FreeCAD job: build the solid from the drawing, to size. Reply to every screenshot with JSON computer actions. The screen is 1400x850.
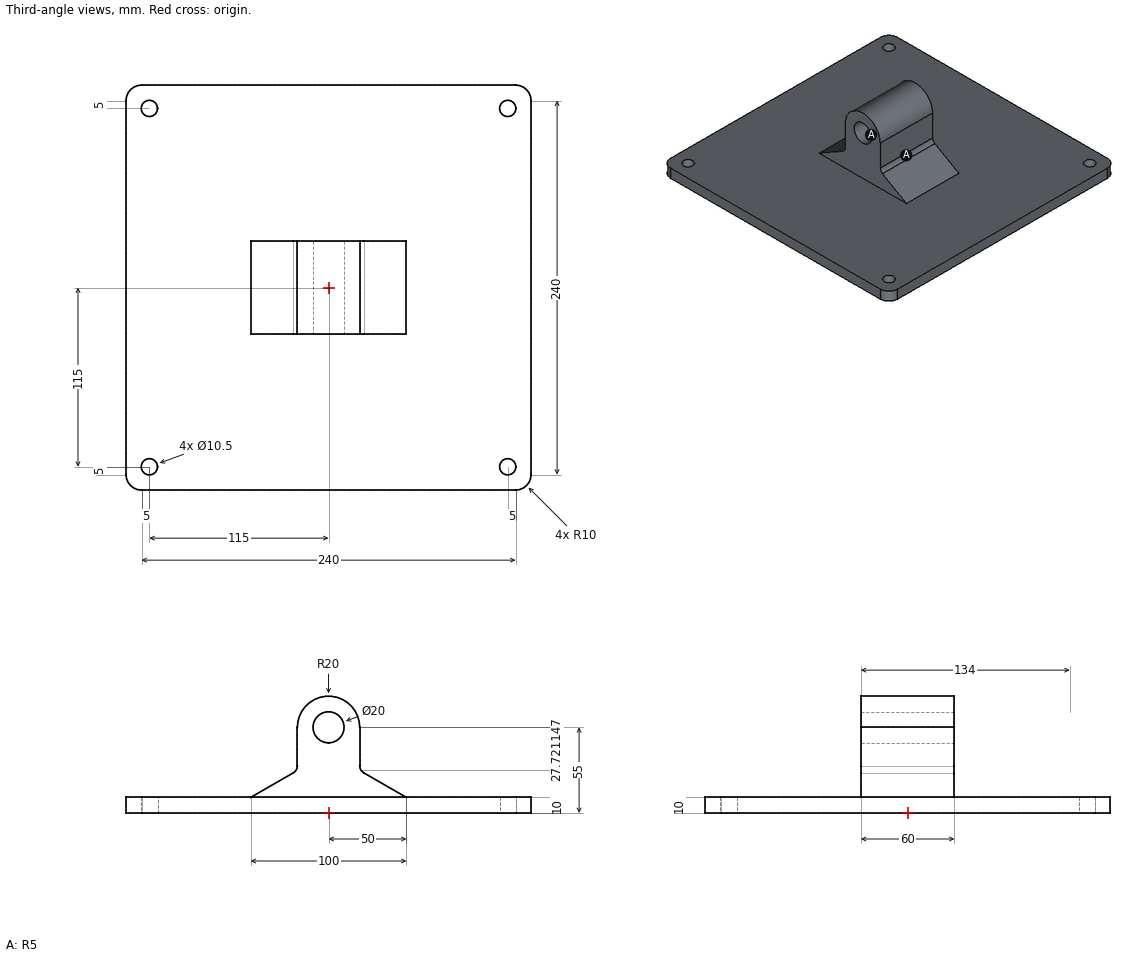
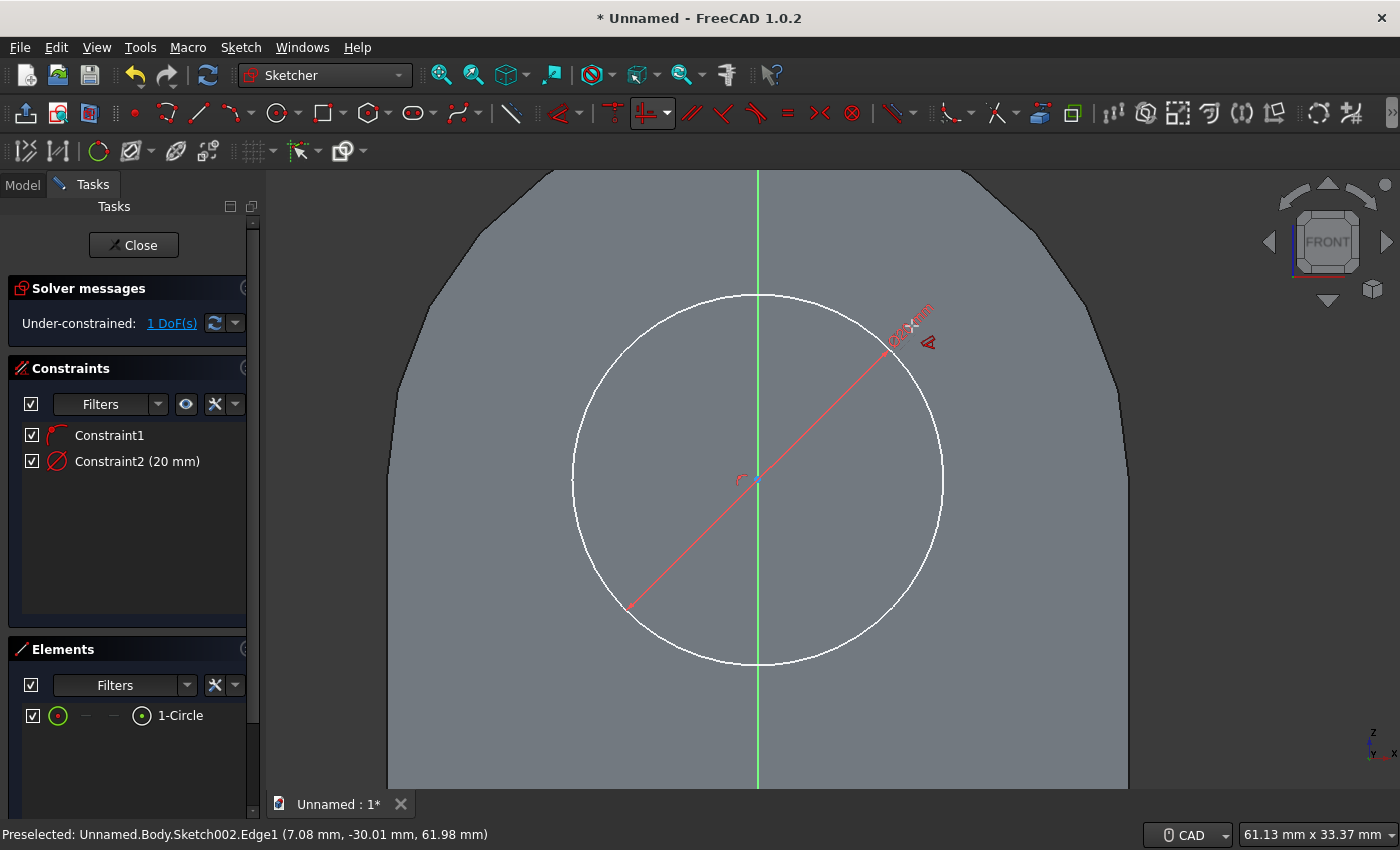
{"action": "left_click", "coordinate": [758, 480]}
{"action": "left_click", "coordinate": [792, 621]}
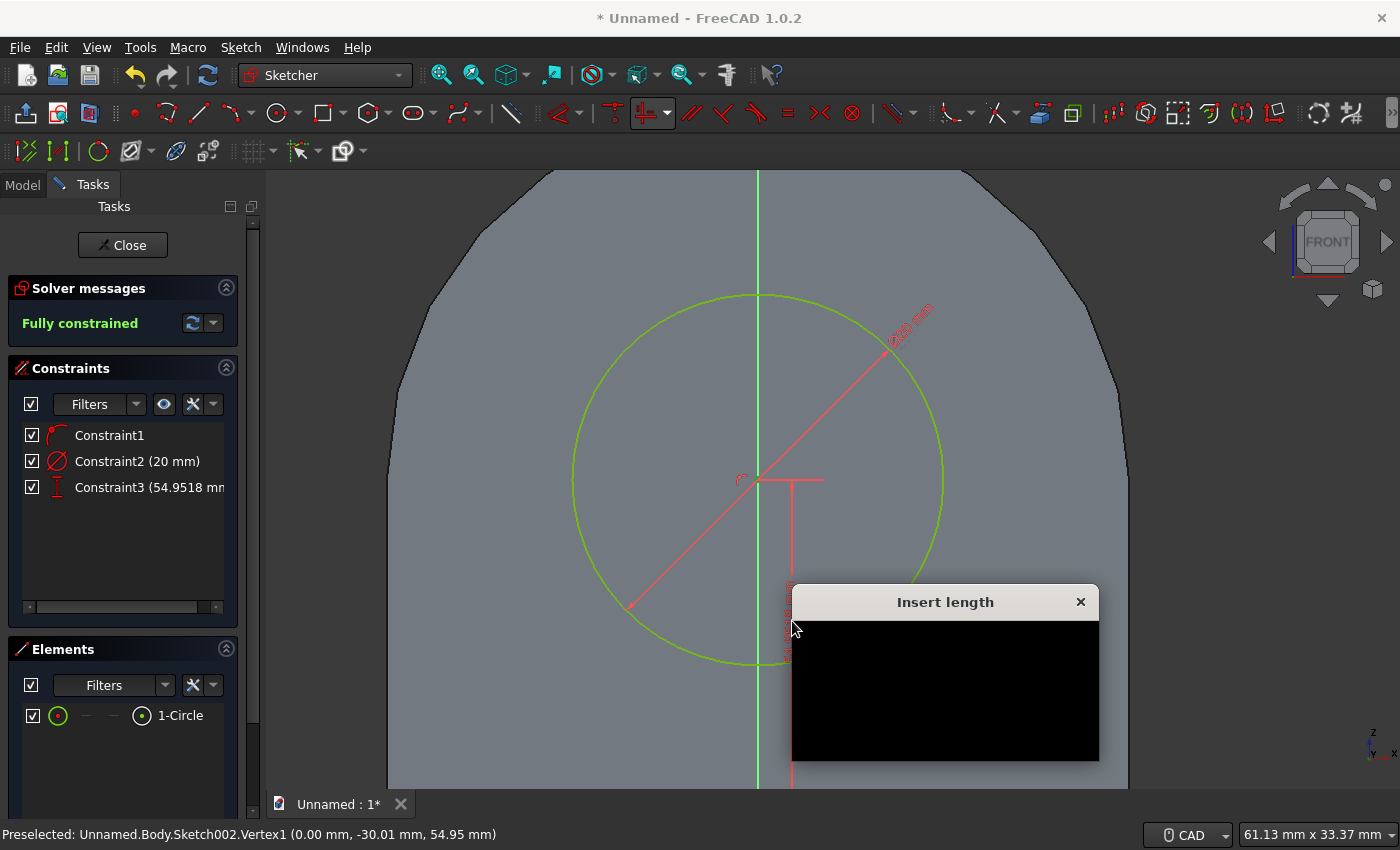
{"action": "type", "text": "55"}
{"action": "key", "text": "Return"}
{"action": "key", "text": "Escape"}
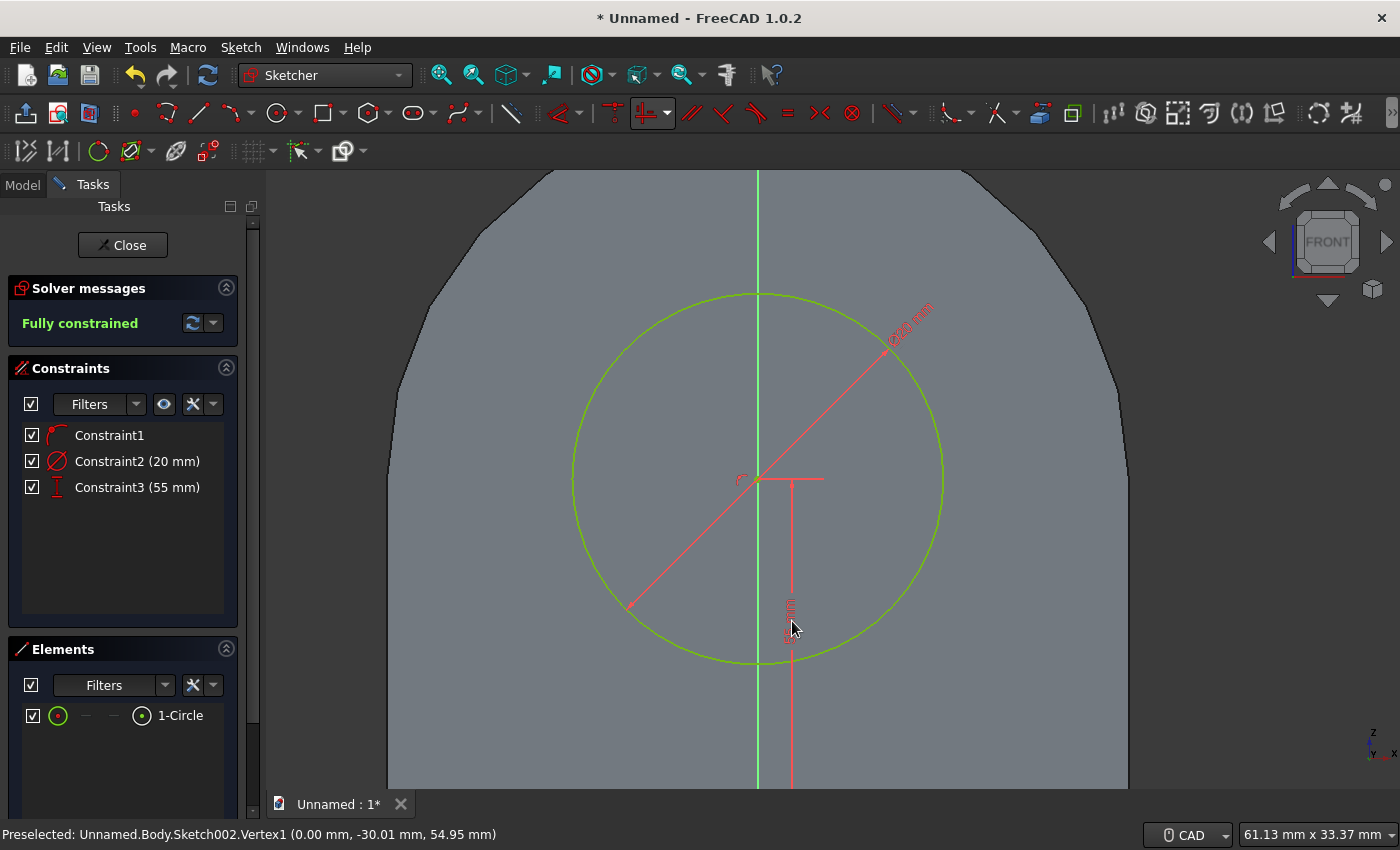
{"action": "left_click", "coordinate": [123, 245]}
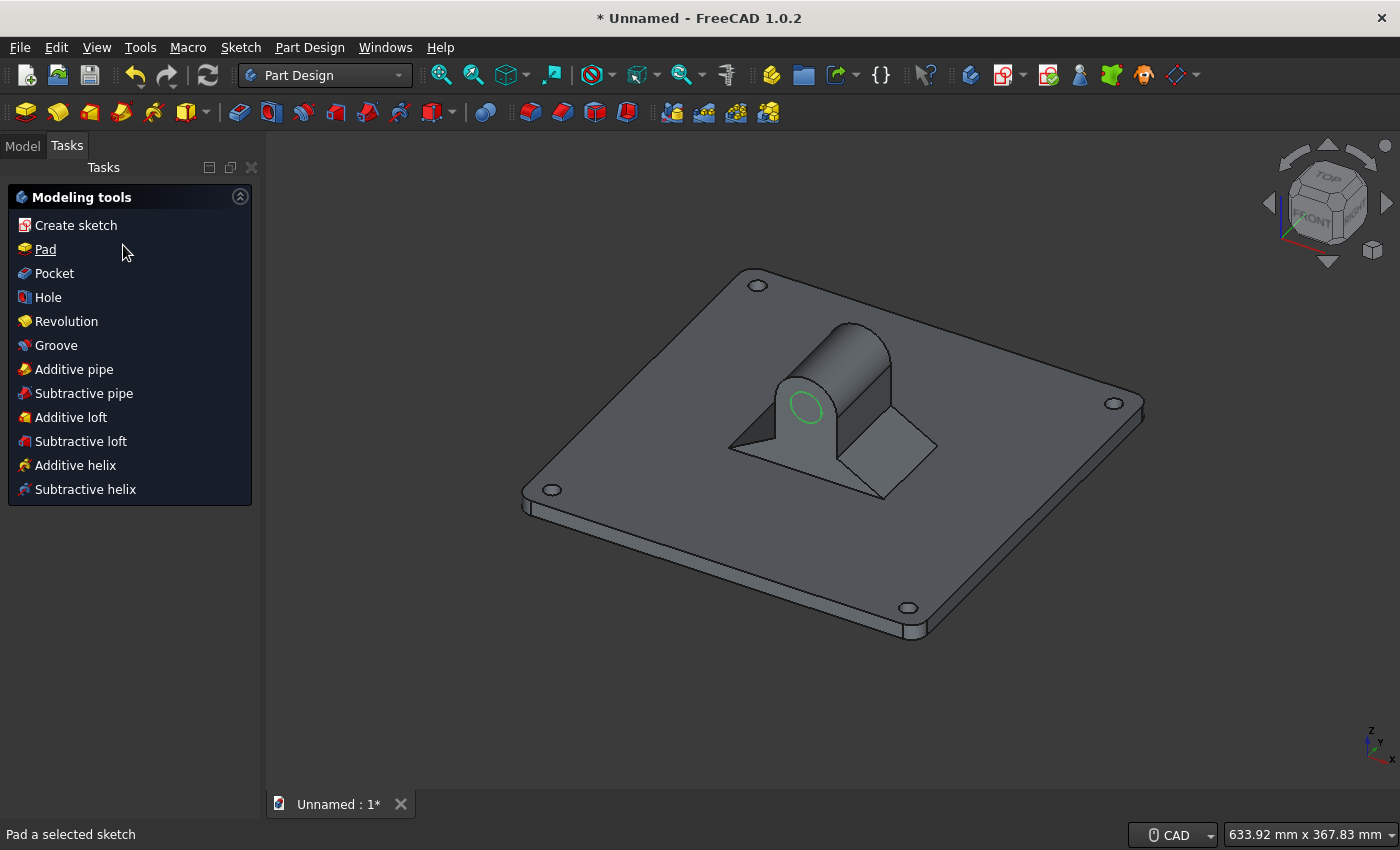
{"action": "left_click", "coordinate": [240, 112]}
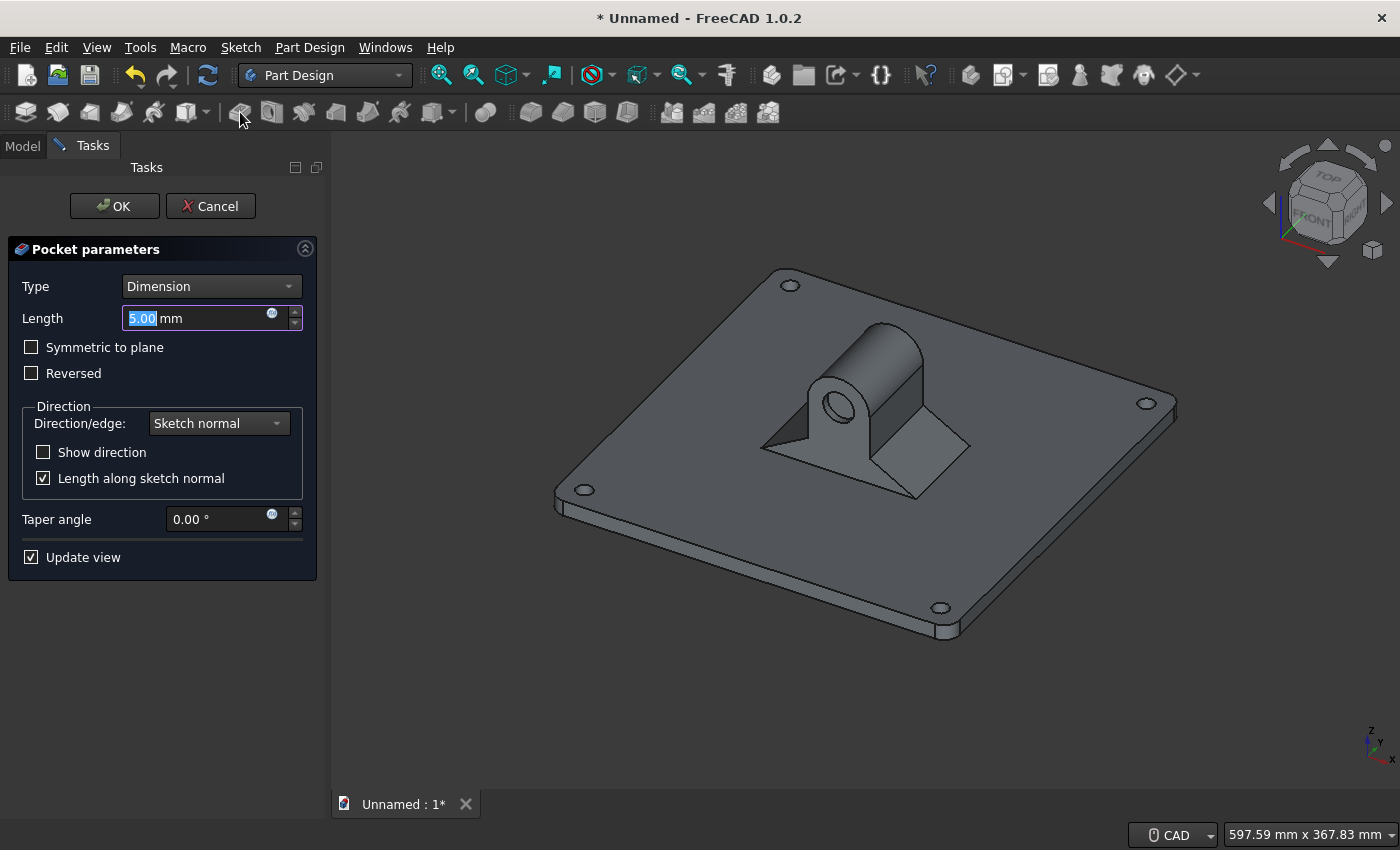
{"action": "type", "text": "134"}
{"action": "key", "text": "Tab"}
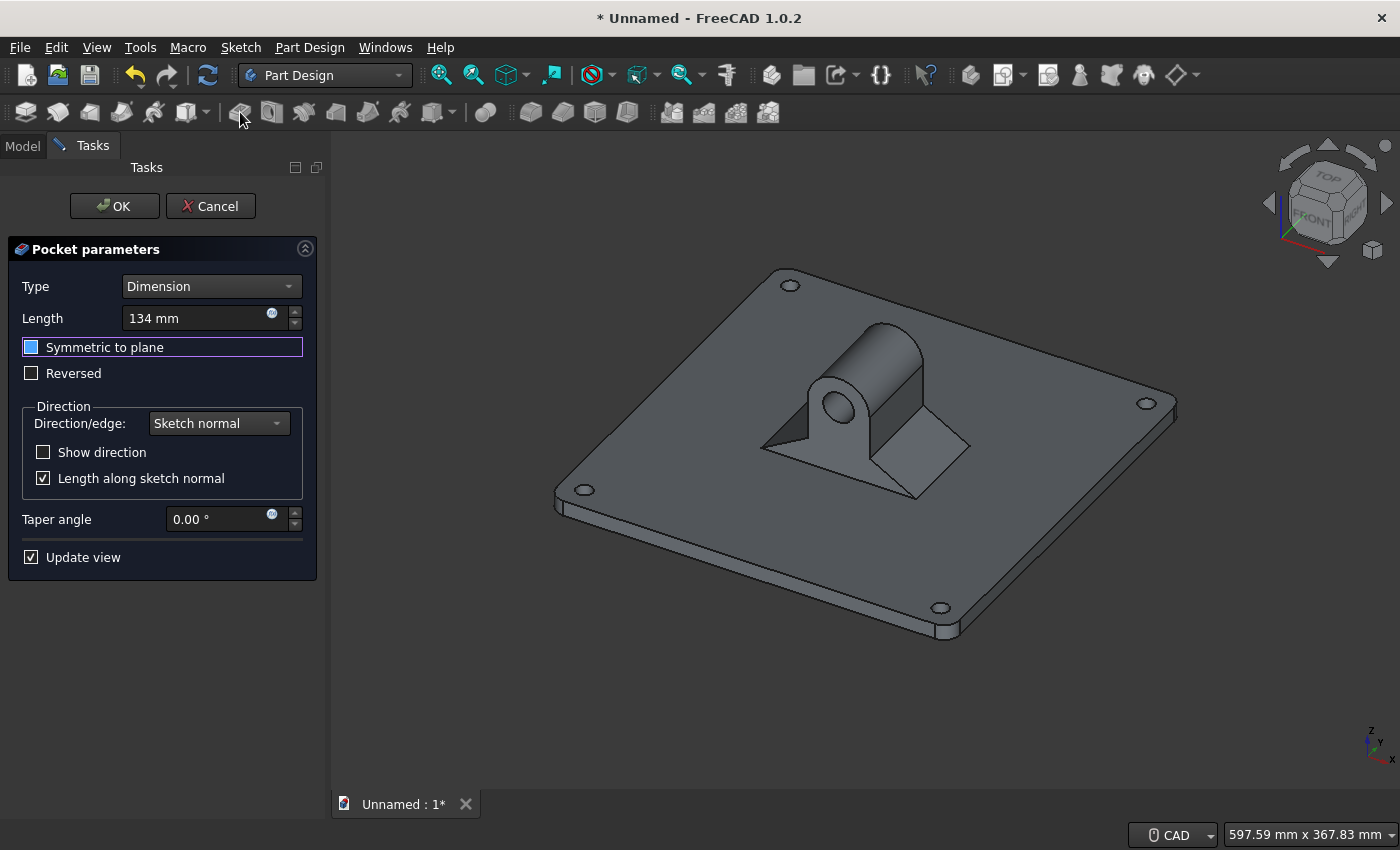
{"action": "left_click", "coordinate": [115, 206]}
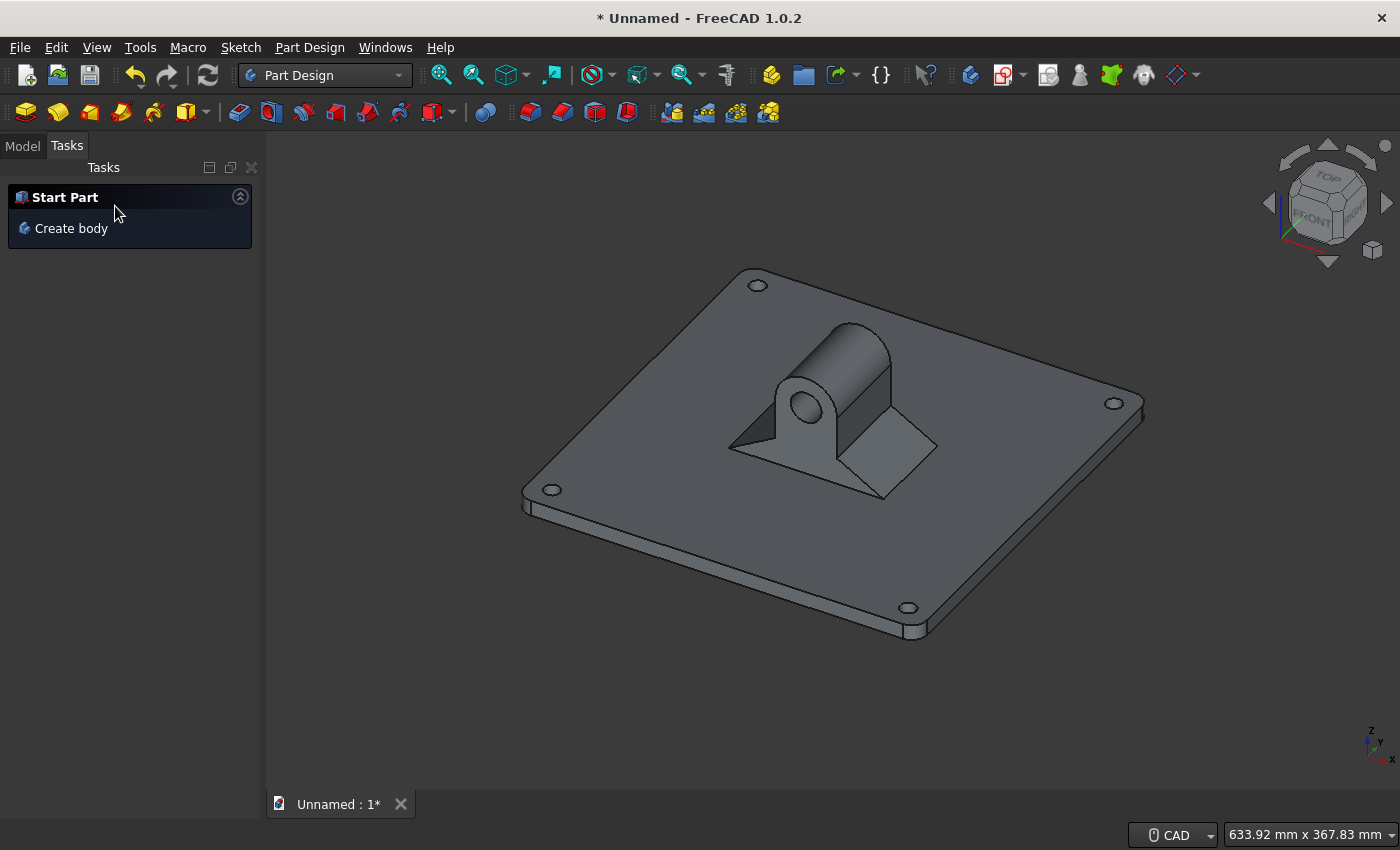
{"action": "key", "text": "0"}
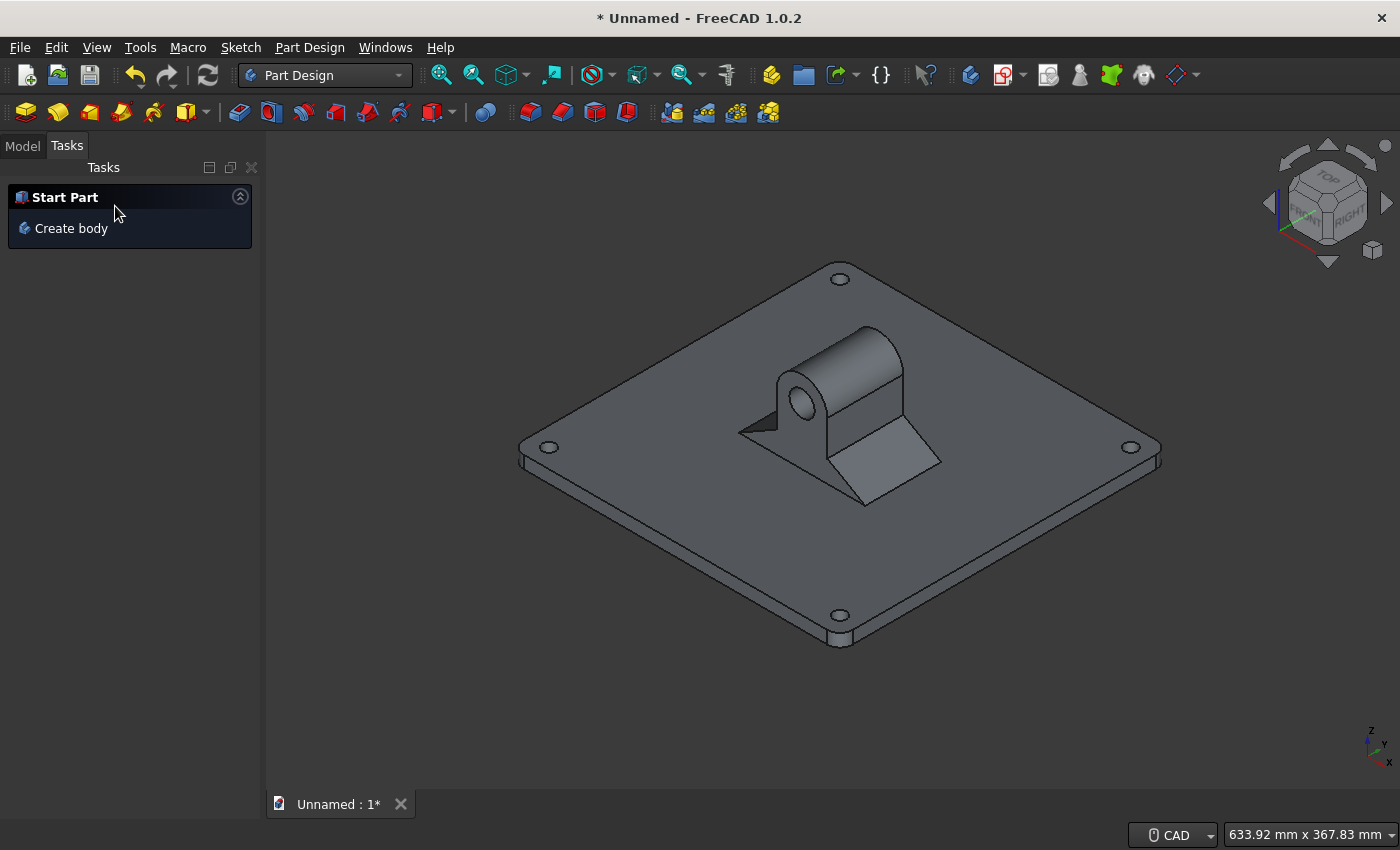
{"action": "key", "text": "2"}